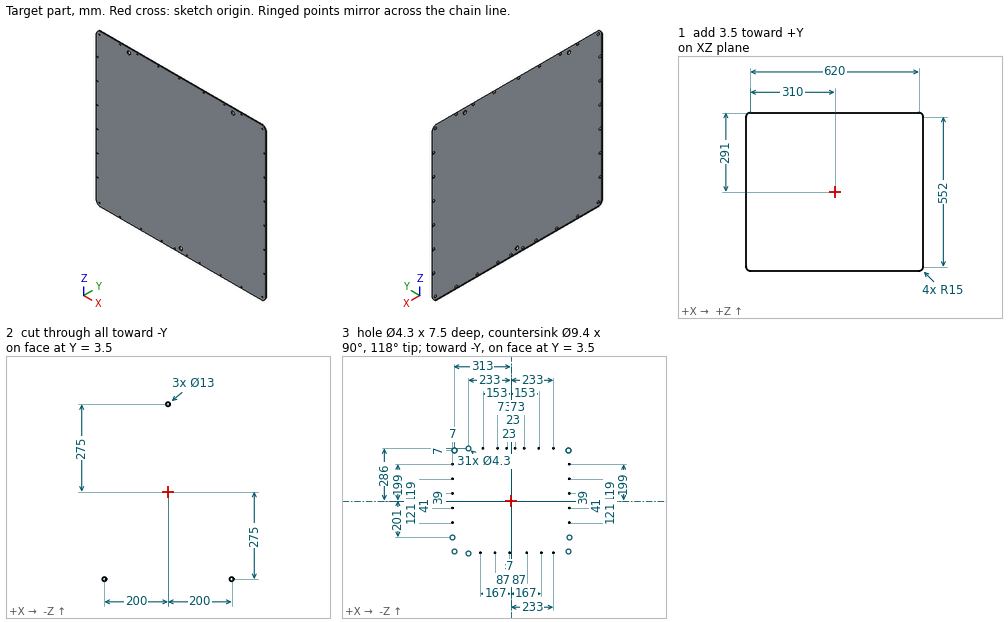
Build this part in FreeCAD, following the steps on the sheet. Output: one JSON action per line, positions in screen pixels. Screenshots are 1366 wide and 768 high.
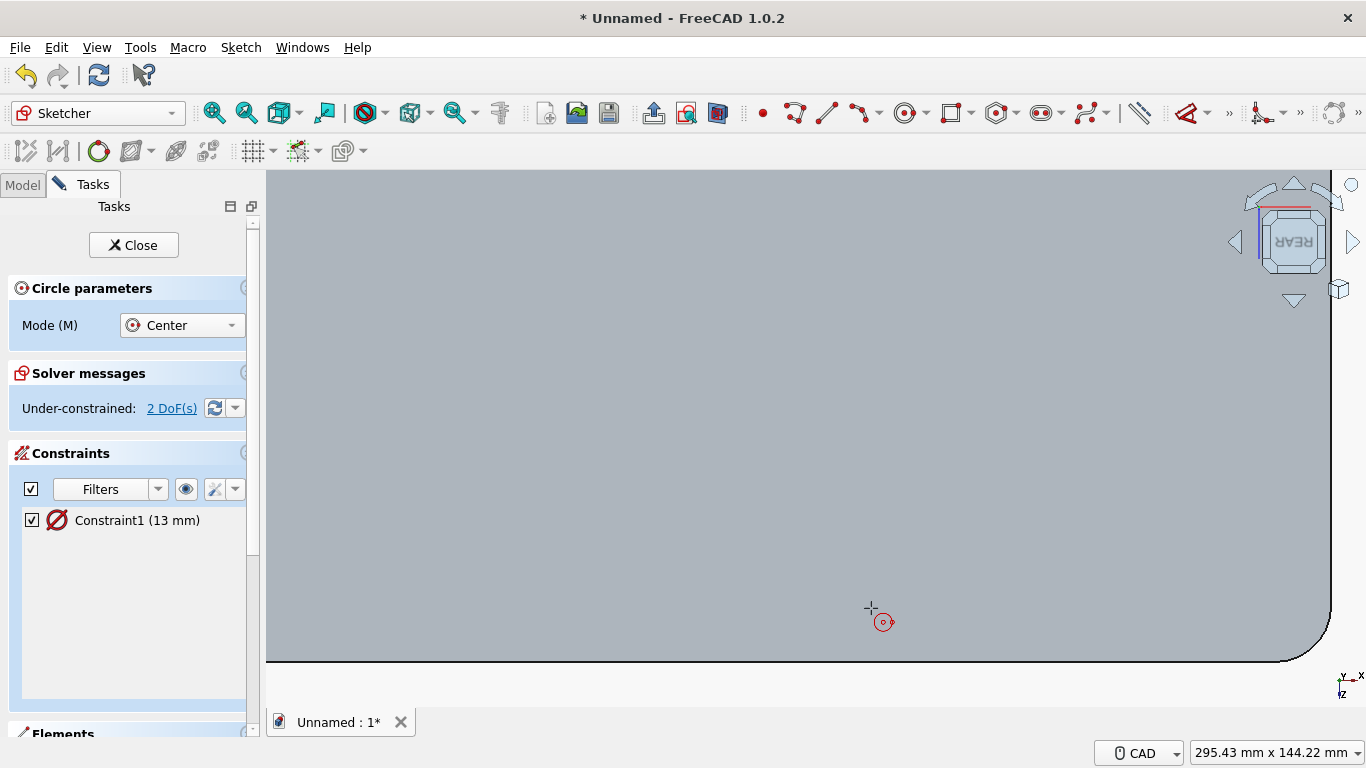
{"action": "scroll", "coordinate": [872, 609], "scroll_direction": "down", "scroll_amount": 9}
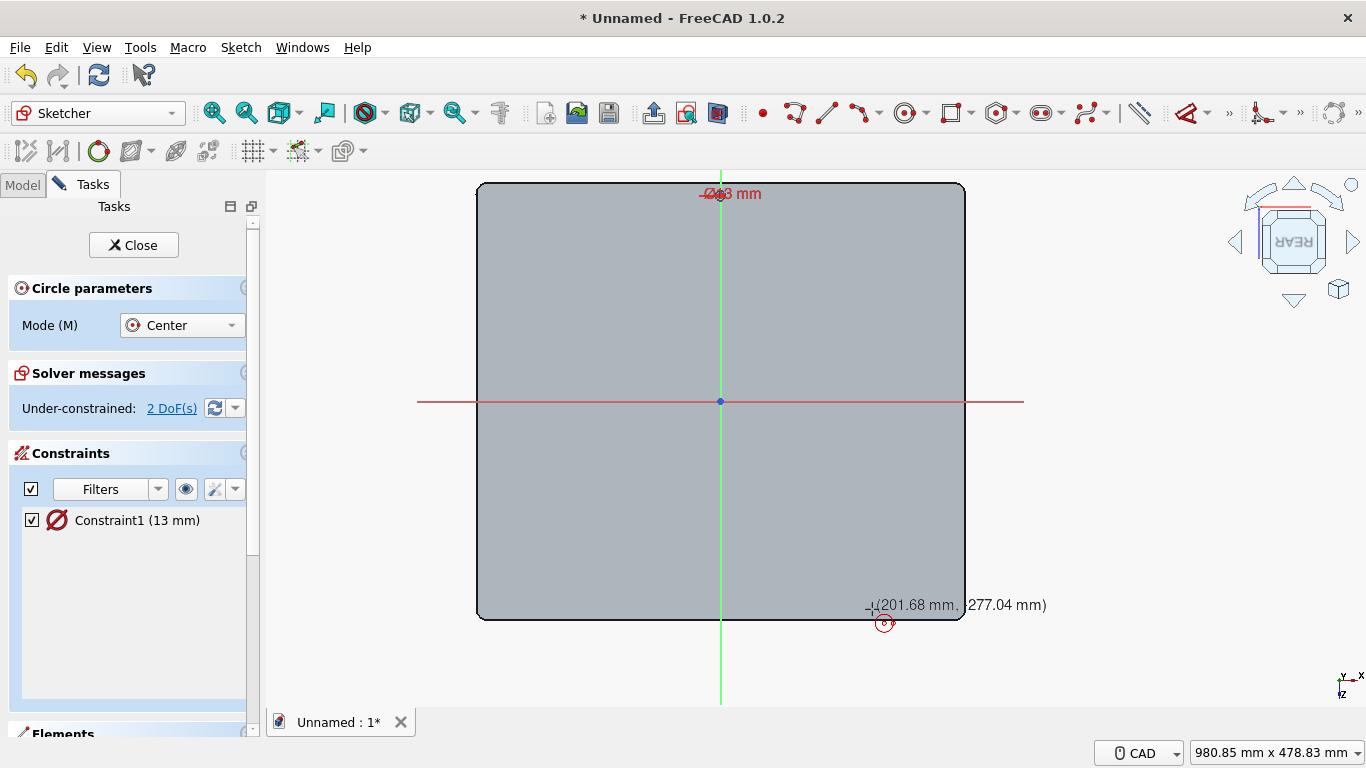
{"action": "left_click", "coordinate": [871, 609]}
{"action": "mouse_move", "coordinate": [874, 606]}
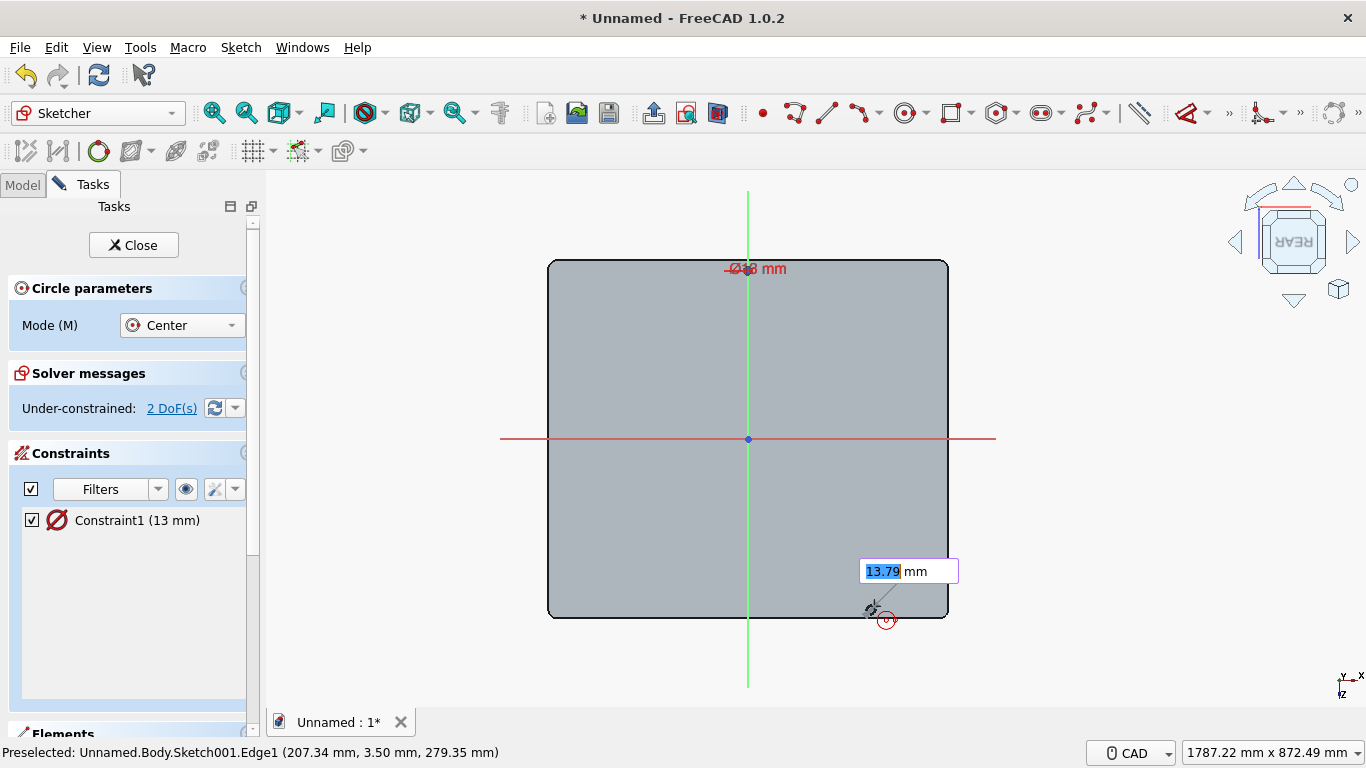
{"action": "type", "text": "13"}
{"action": "key", "text": "Return"}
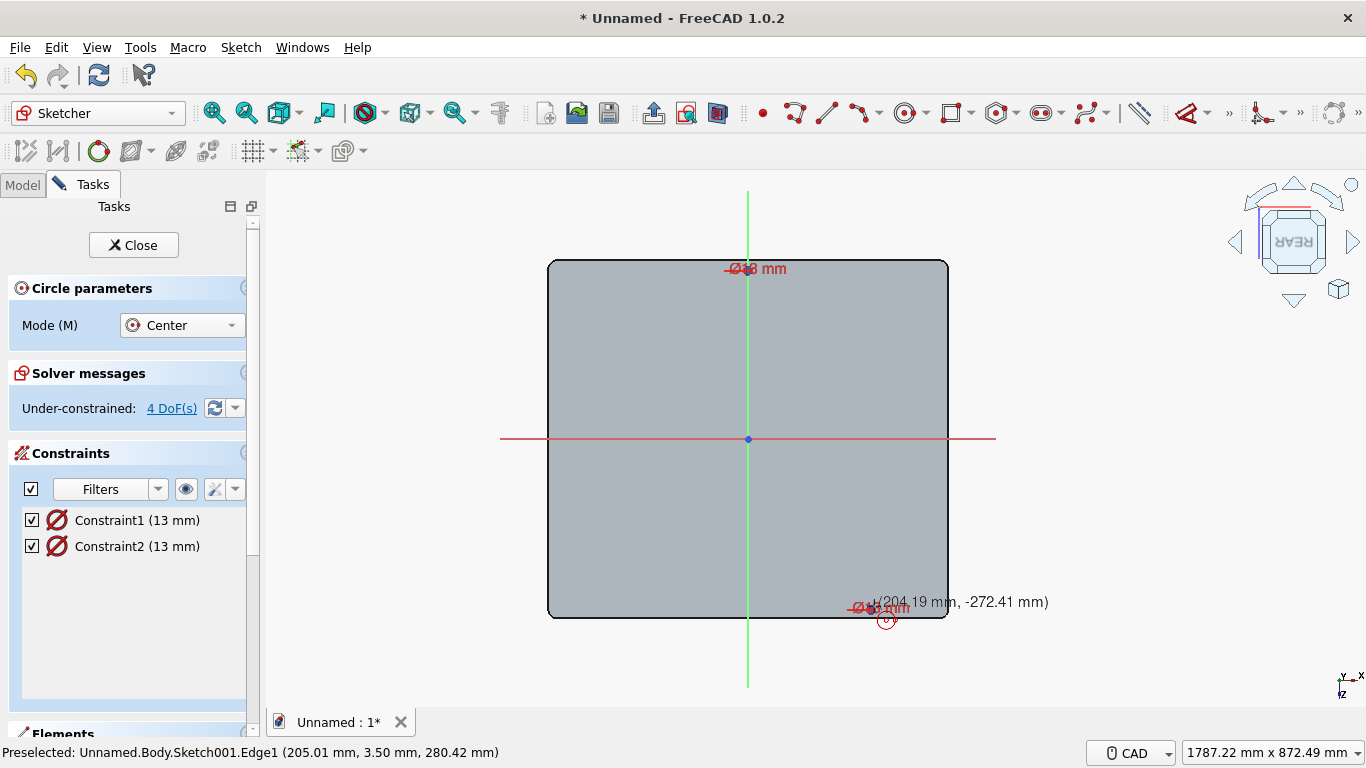
{"action": "scroll", "coordinate": [625, 609], "scroll_direction": "up", "scroll_amount": 9}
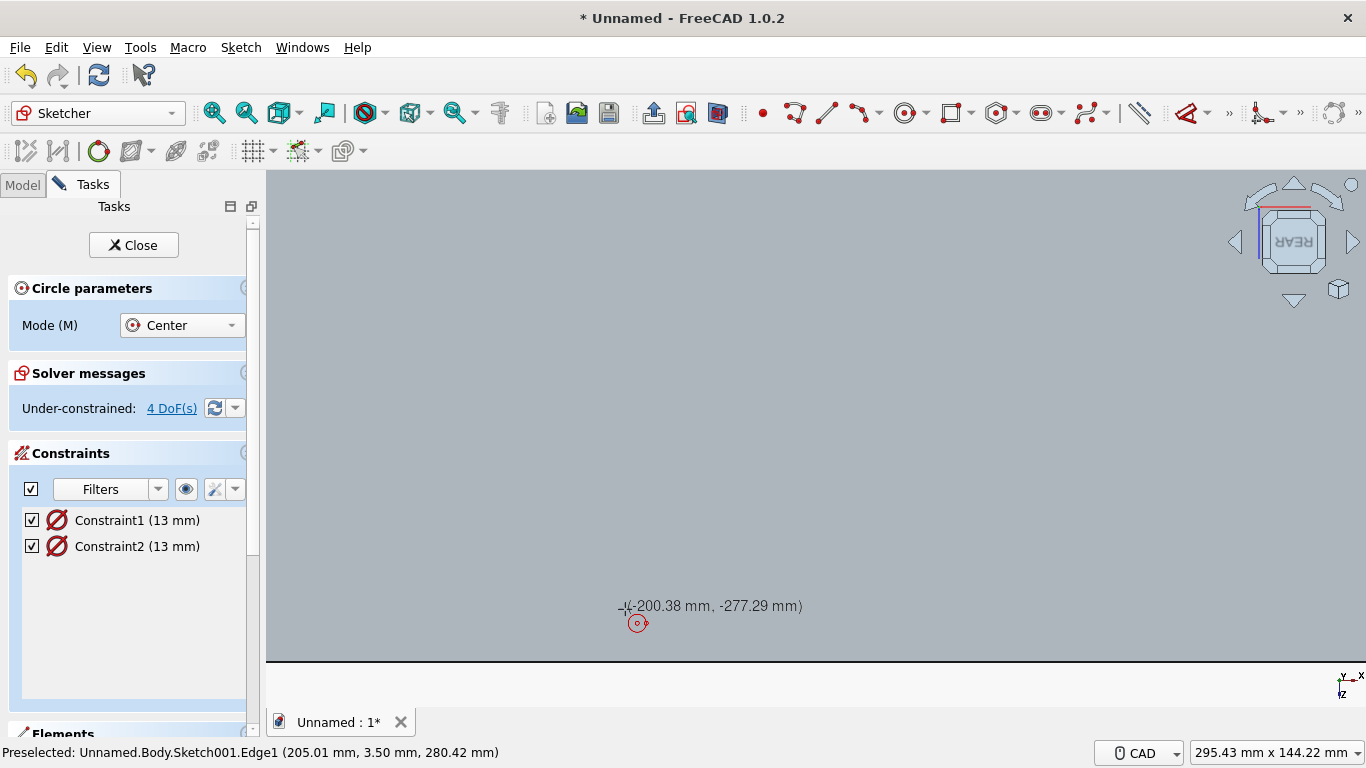
{"action": "scroll", "coordinate": [624, 609], "scroll_direction": "down", "scroll_amount": 9}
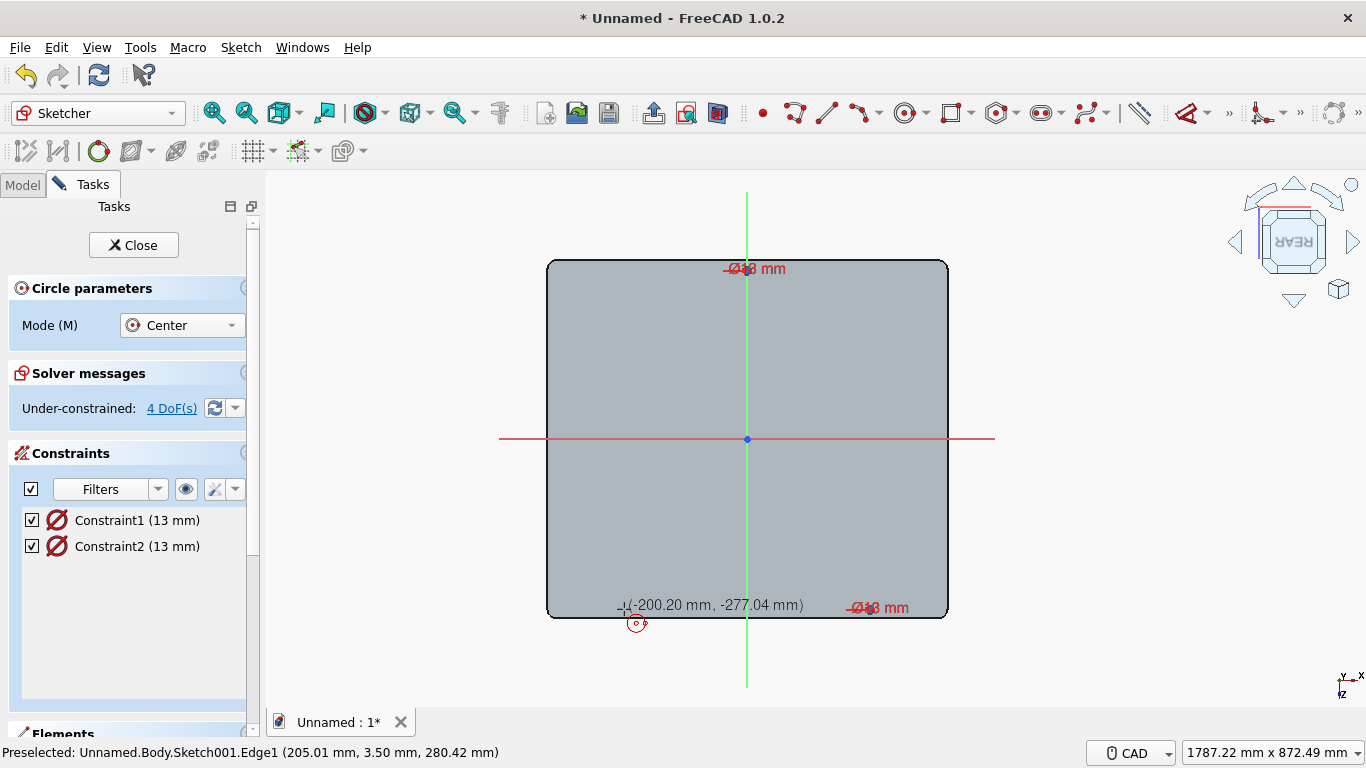
{"action": "left_click", "coordinate": [624, 609]}
{"action": "mouse_move", "coordinate": [627, 606]}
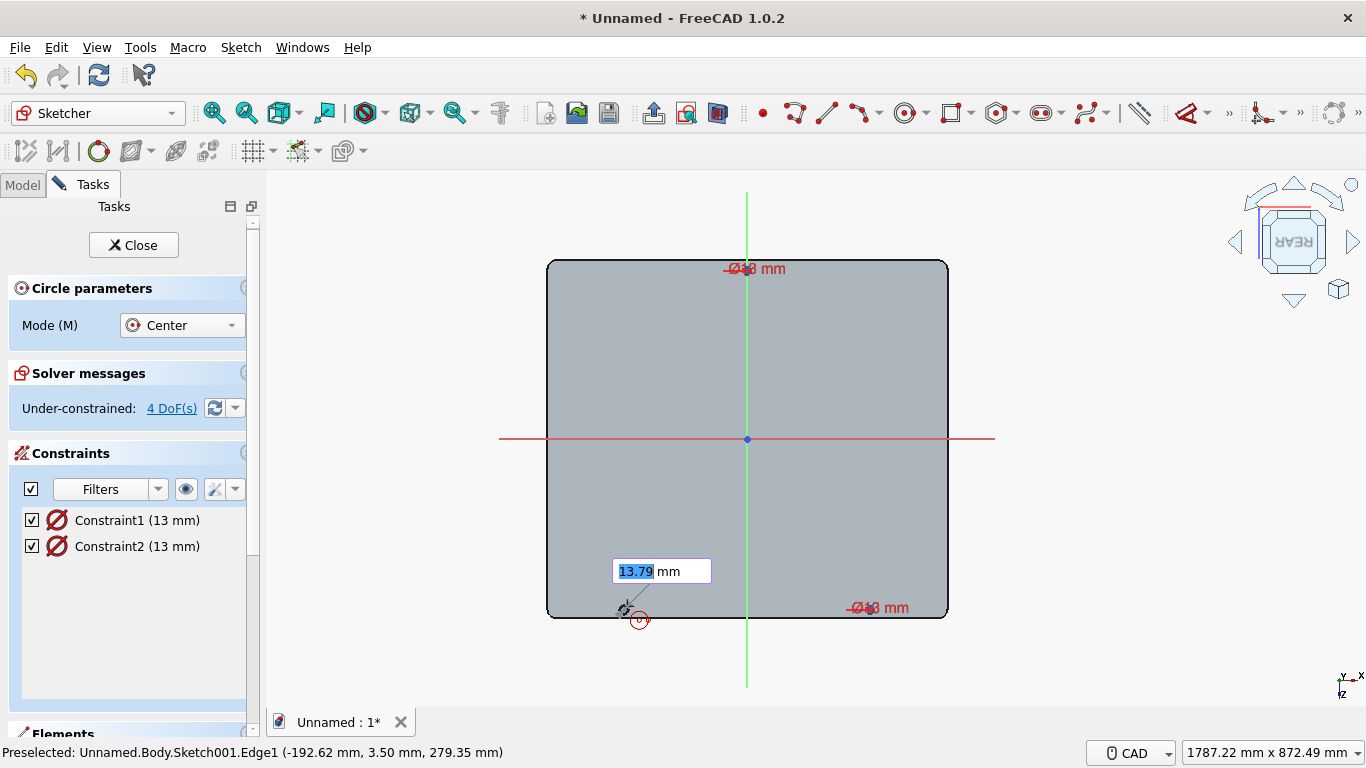
{"action": "type", "text": "13"}
{"action": "key", "text": "Return"}
{"action": "key", "text": "Escape"}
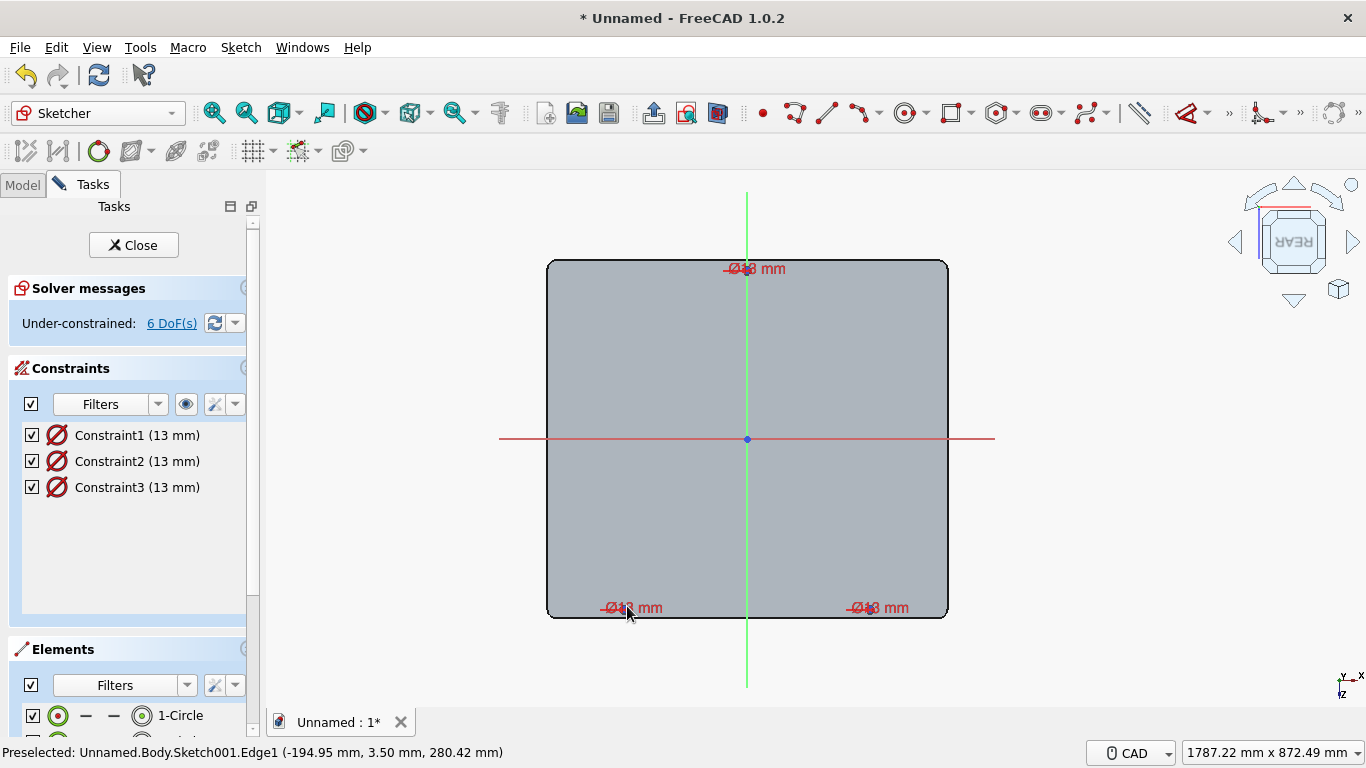
{"action": "left_click", "coordinate": [747, 271]}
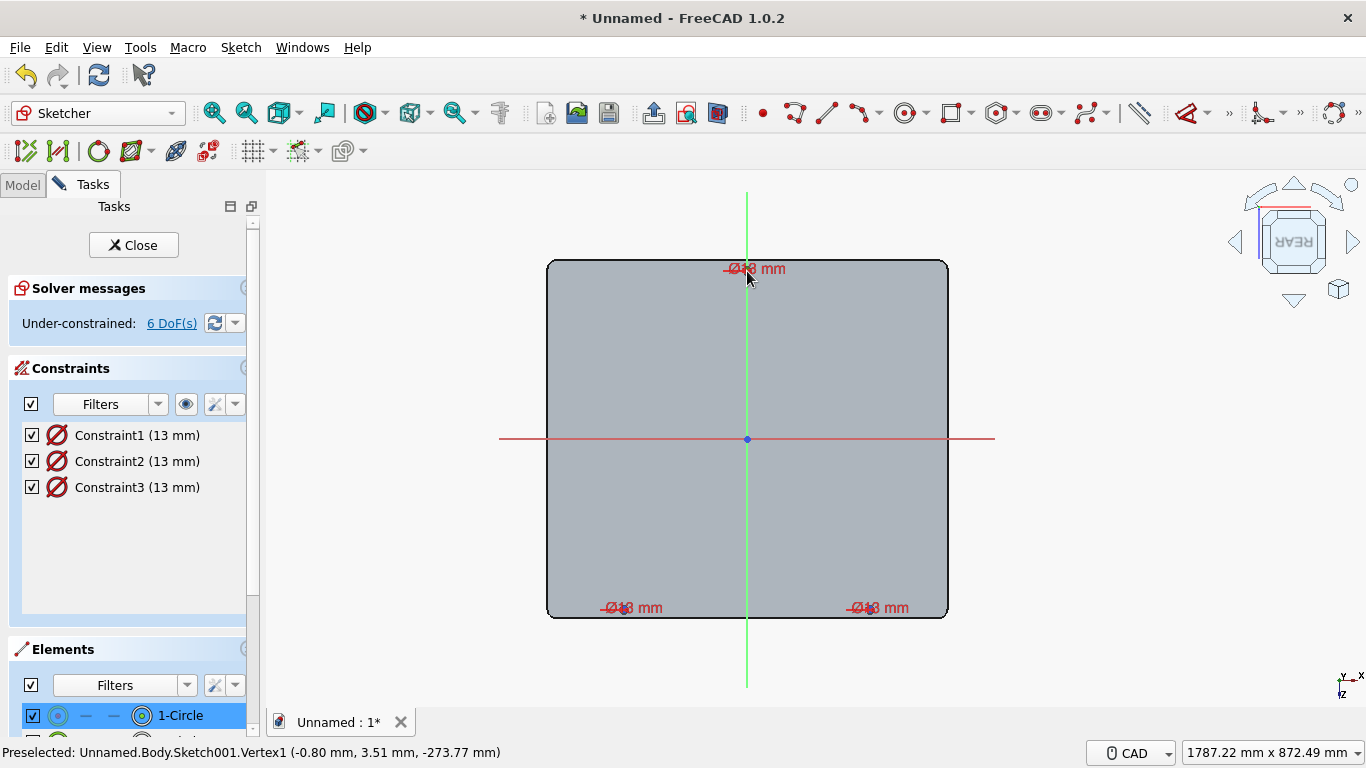
{"action": "left_click", "coordinate": [747, 645]}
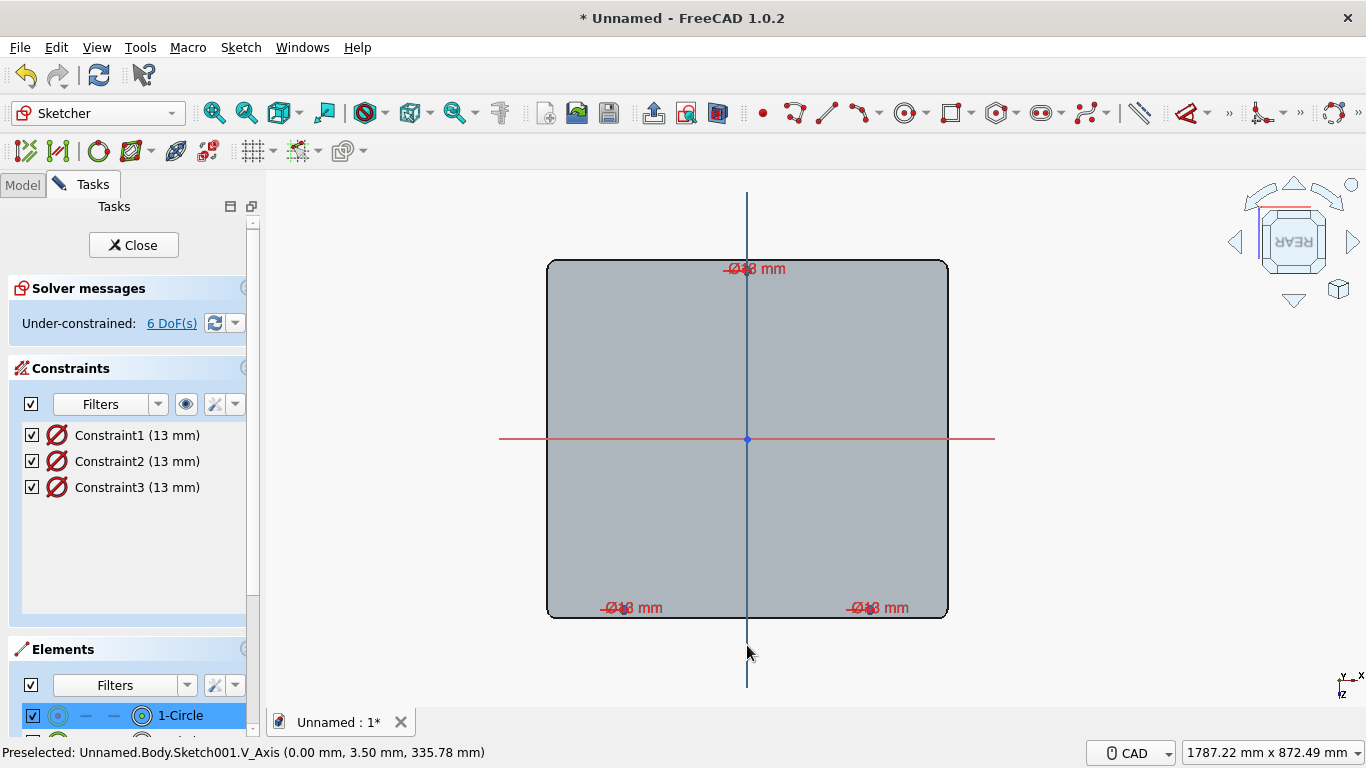
{"action": "key", "text": "c"}